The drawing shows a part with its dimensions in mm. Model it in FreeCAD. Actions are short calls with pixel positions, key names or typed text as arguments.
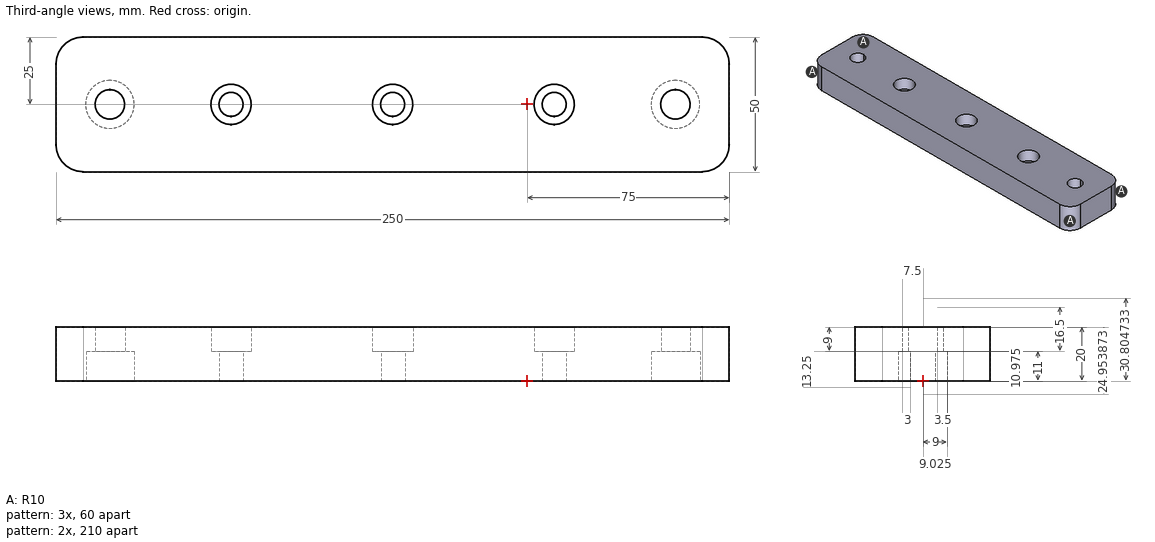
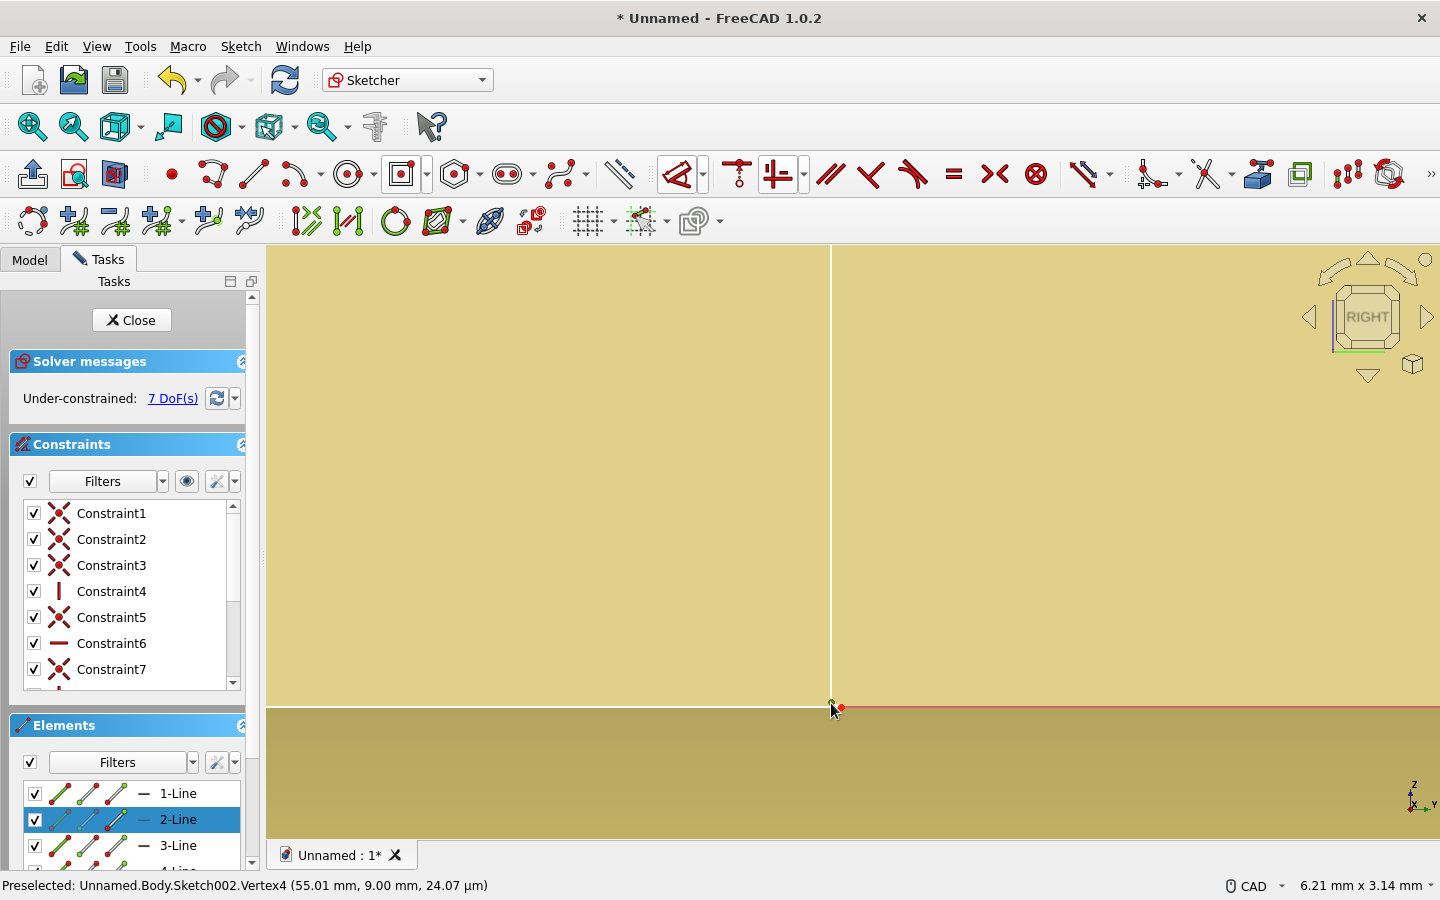
key(l)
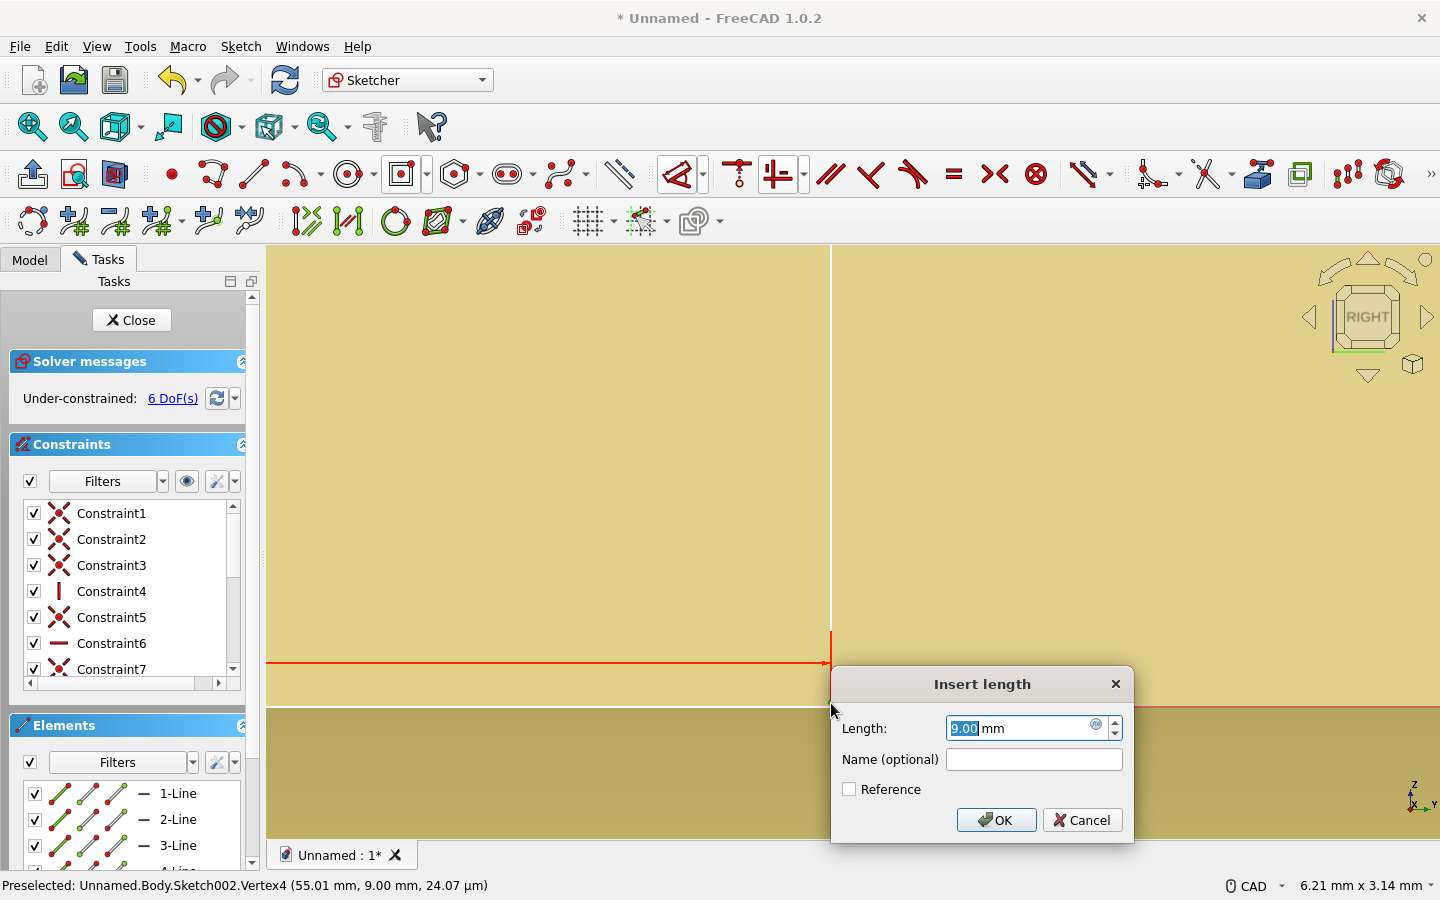
text(9)
key(Return)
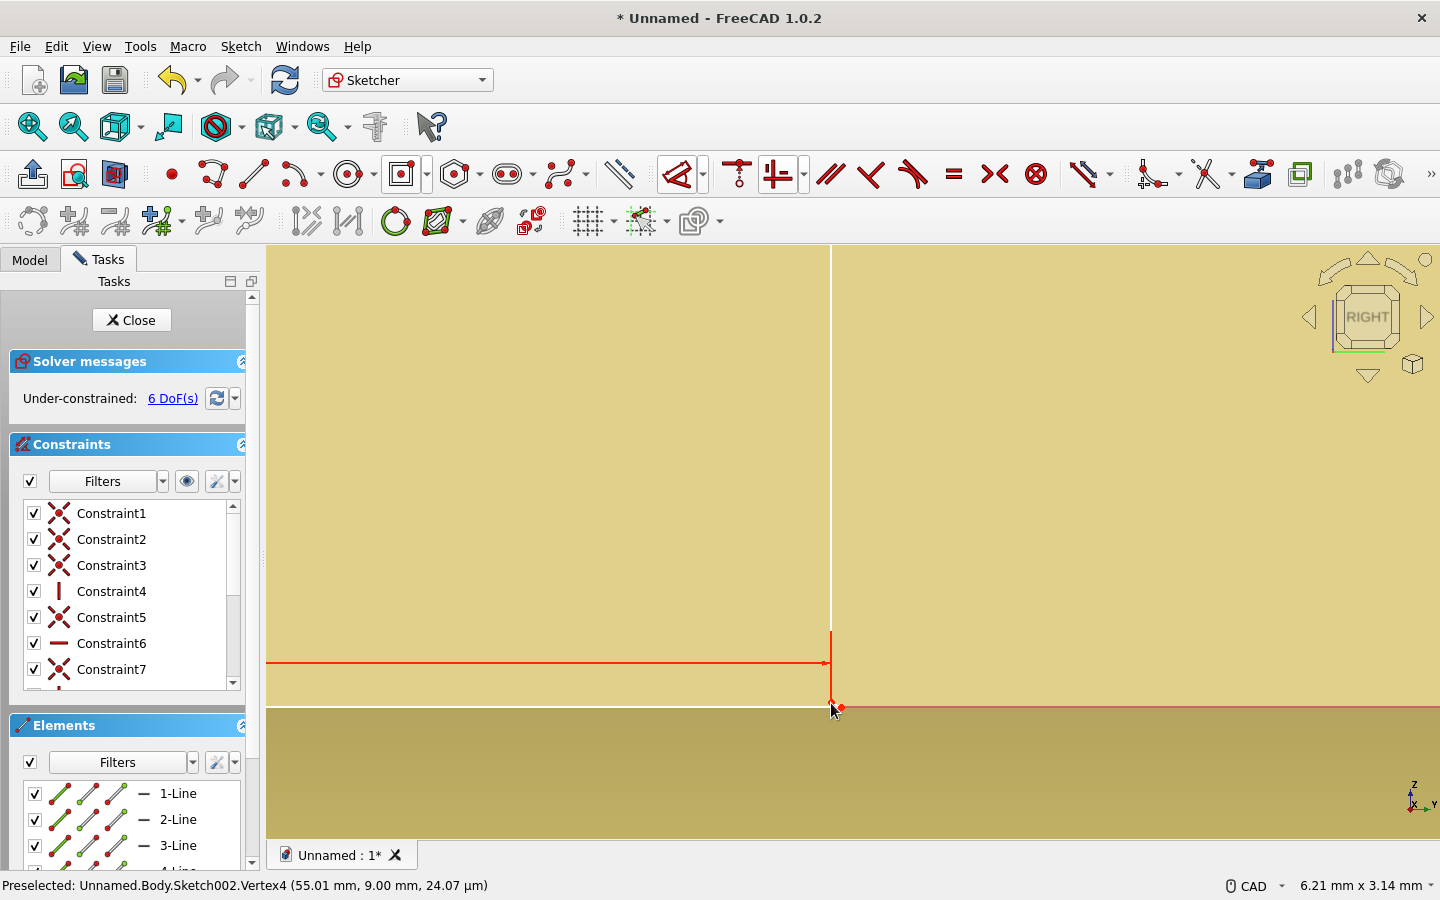
scroll(836, 720, down, 14)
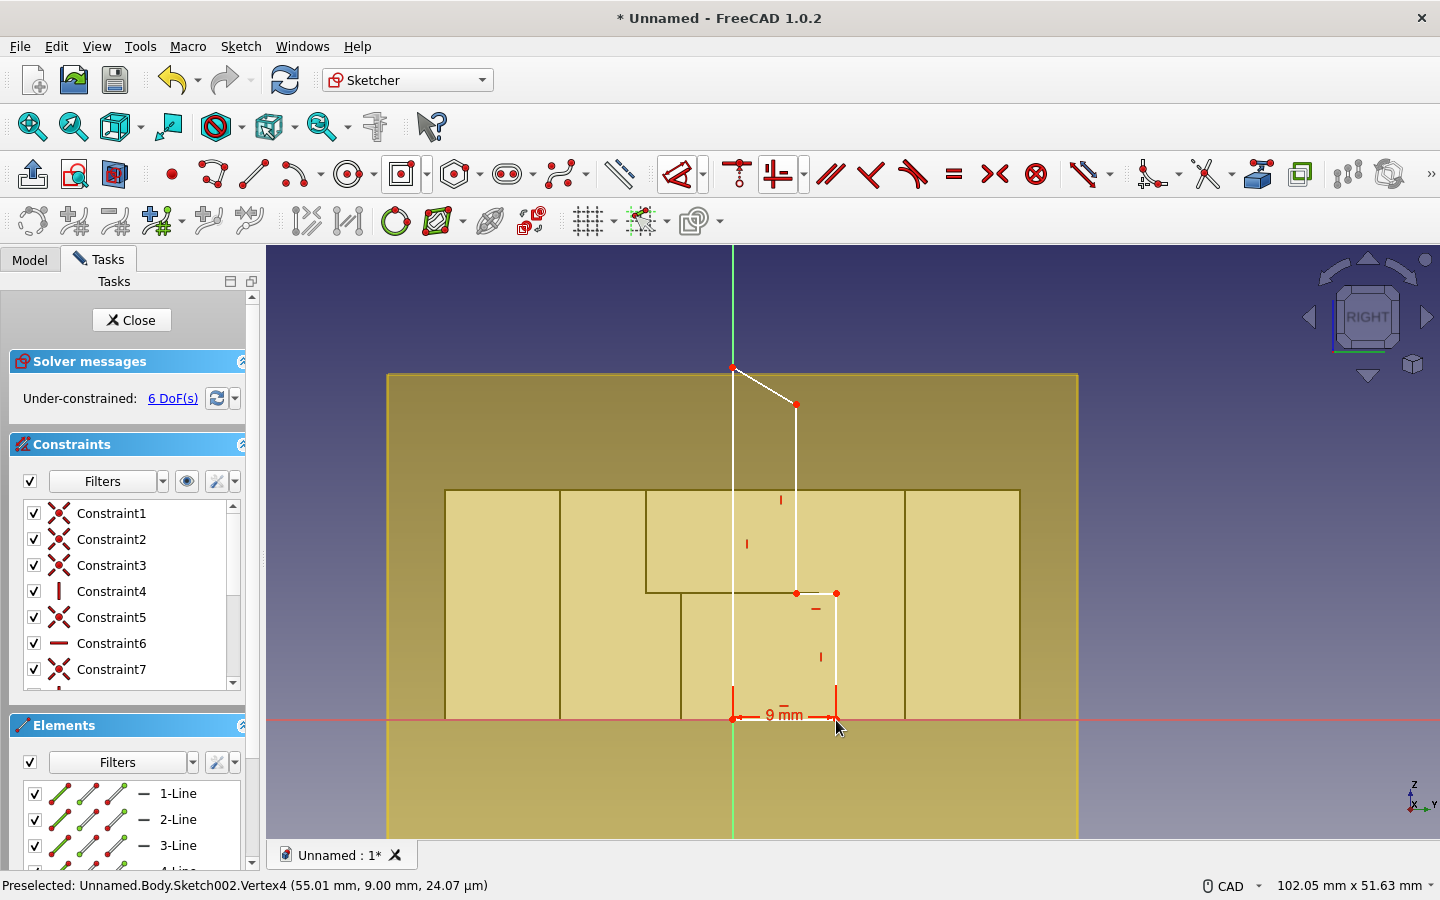
click(824, 594)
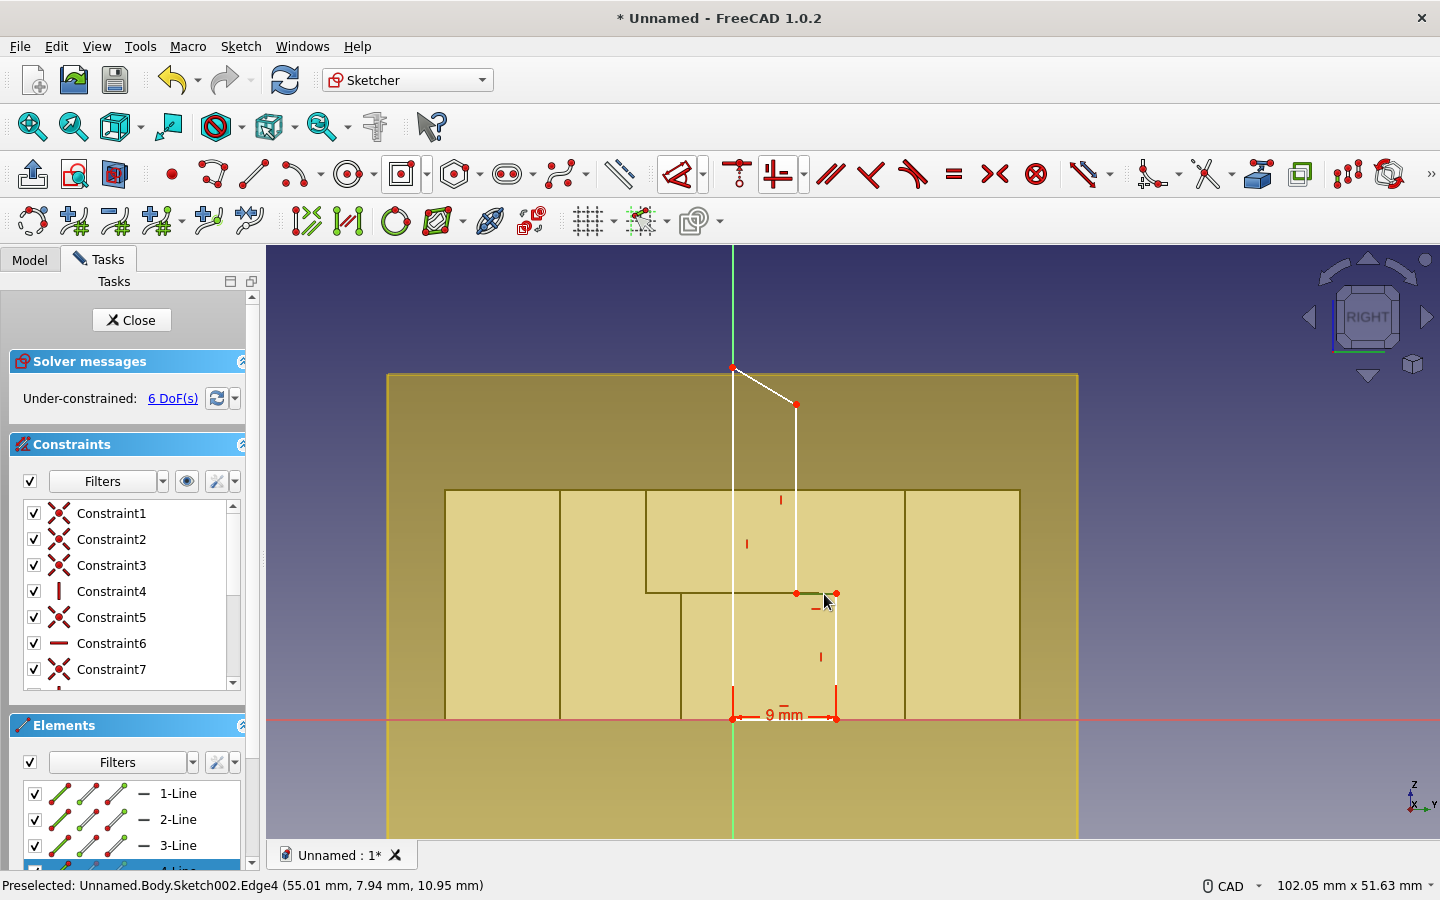
key(l)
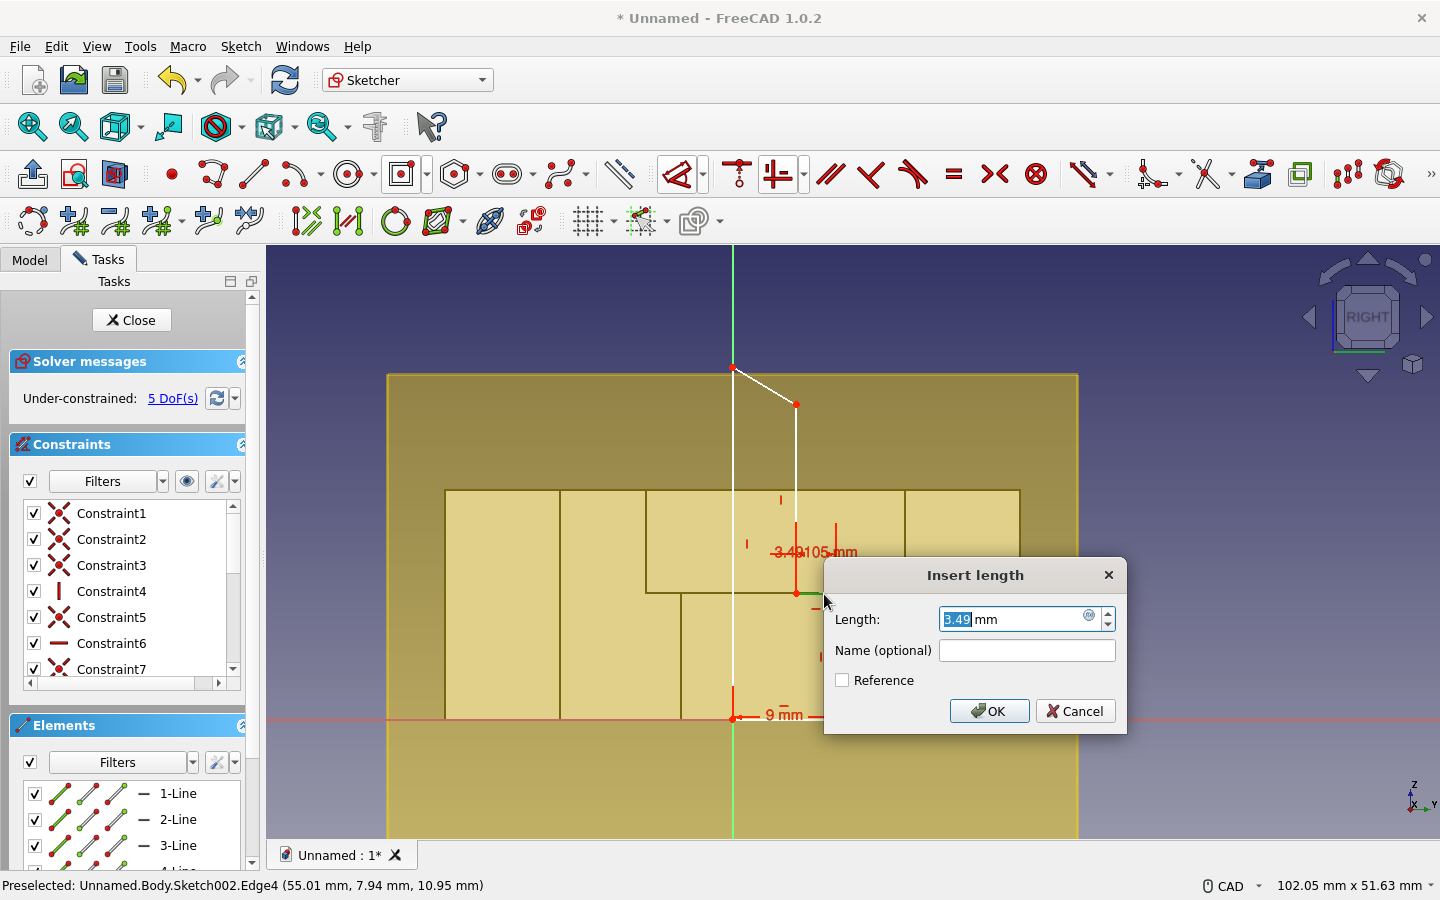
text(3.5)
key(Return)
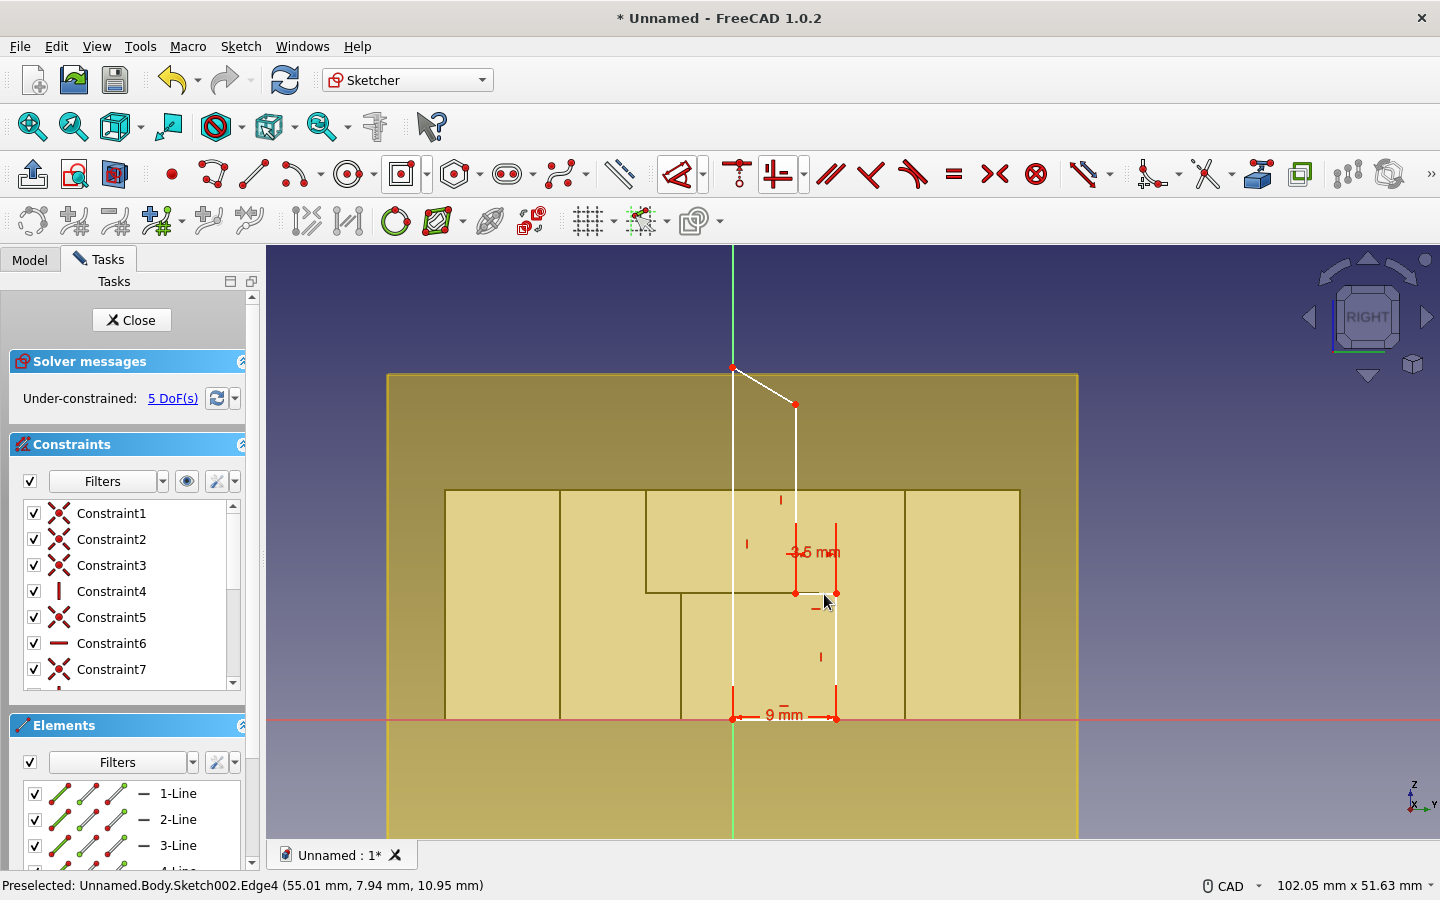
click(836, 594)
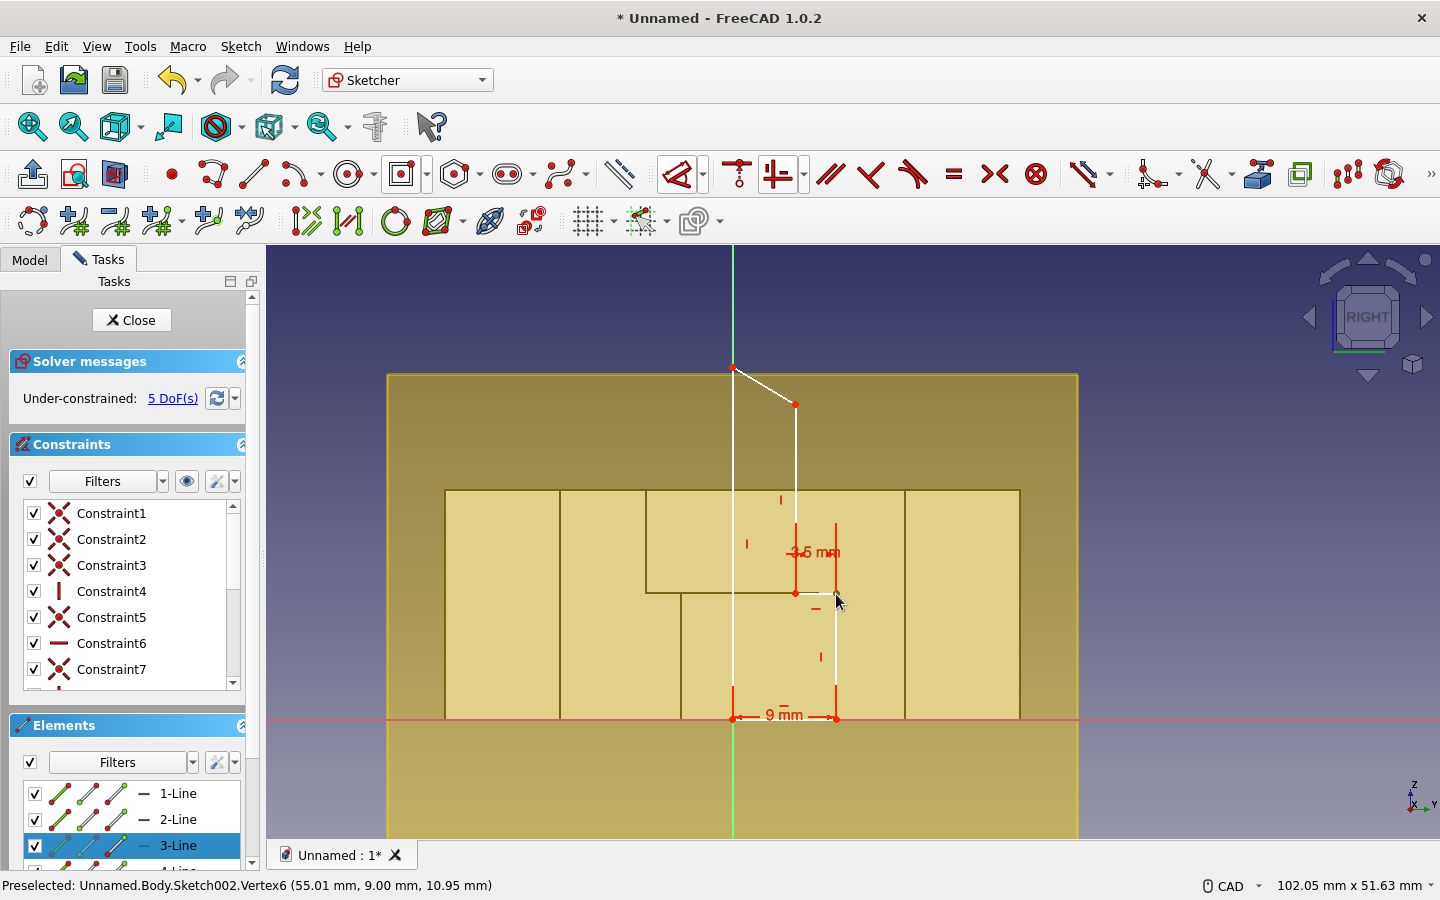
key(i)